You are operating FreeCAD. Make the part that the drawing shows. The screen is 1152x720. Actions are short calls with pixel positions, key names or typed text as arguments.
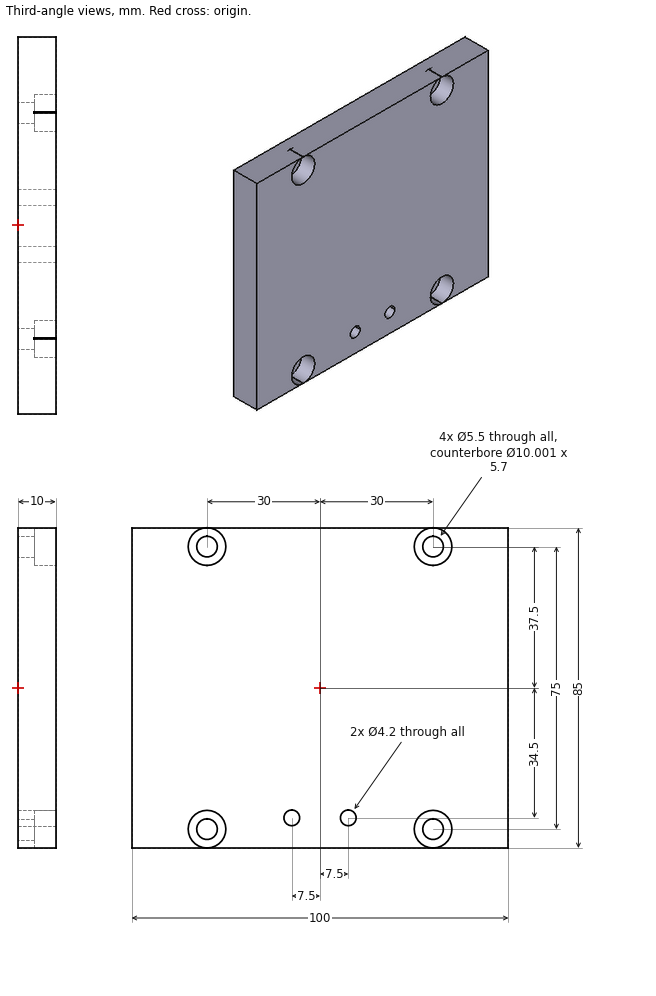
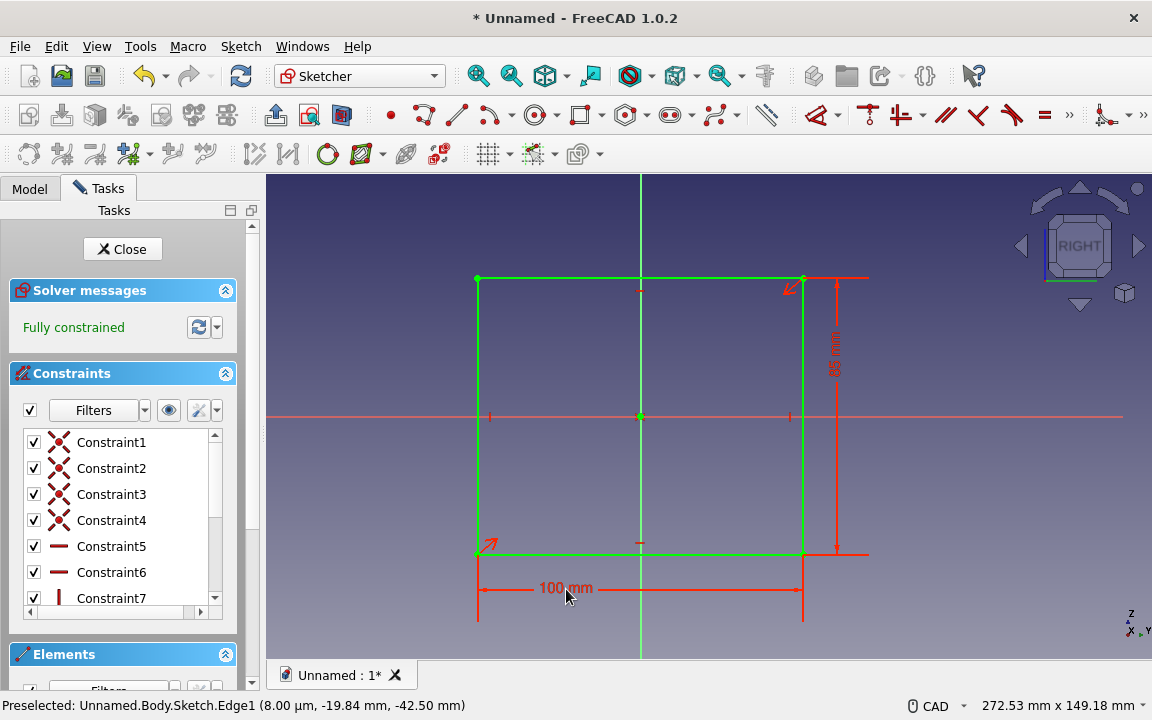
click(123, 249)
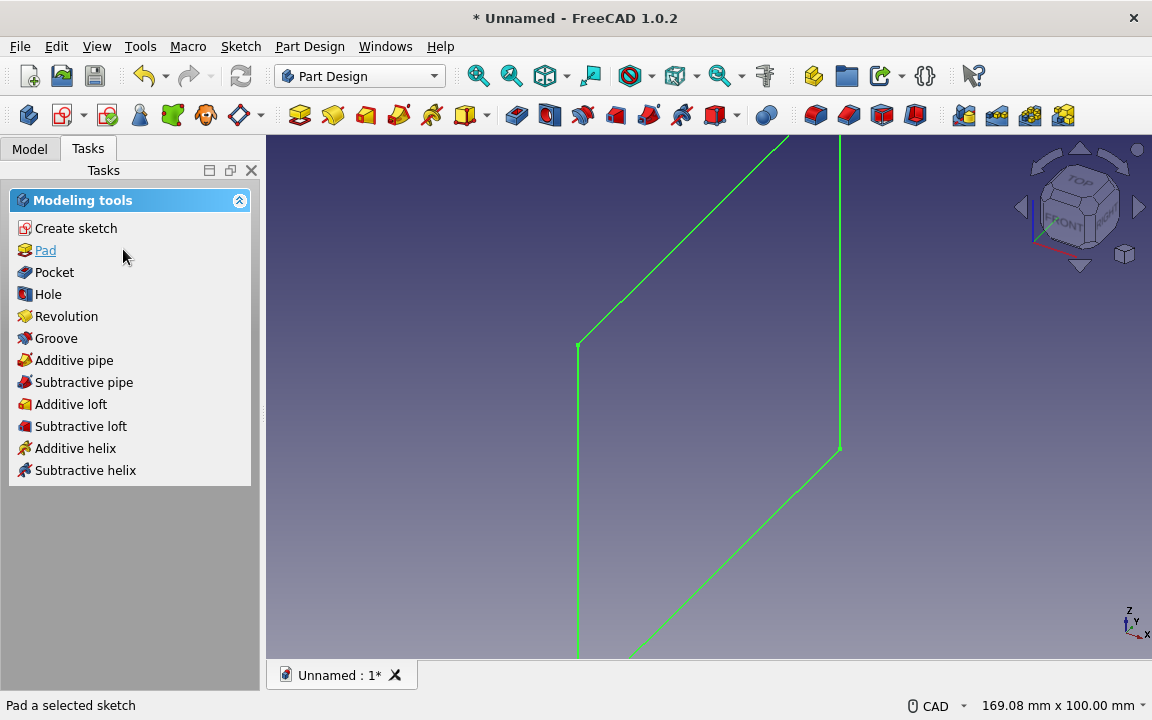
click(300, 116)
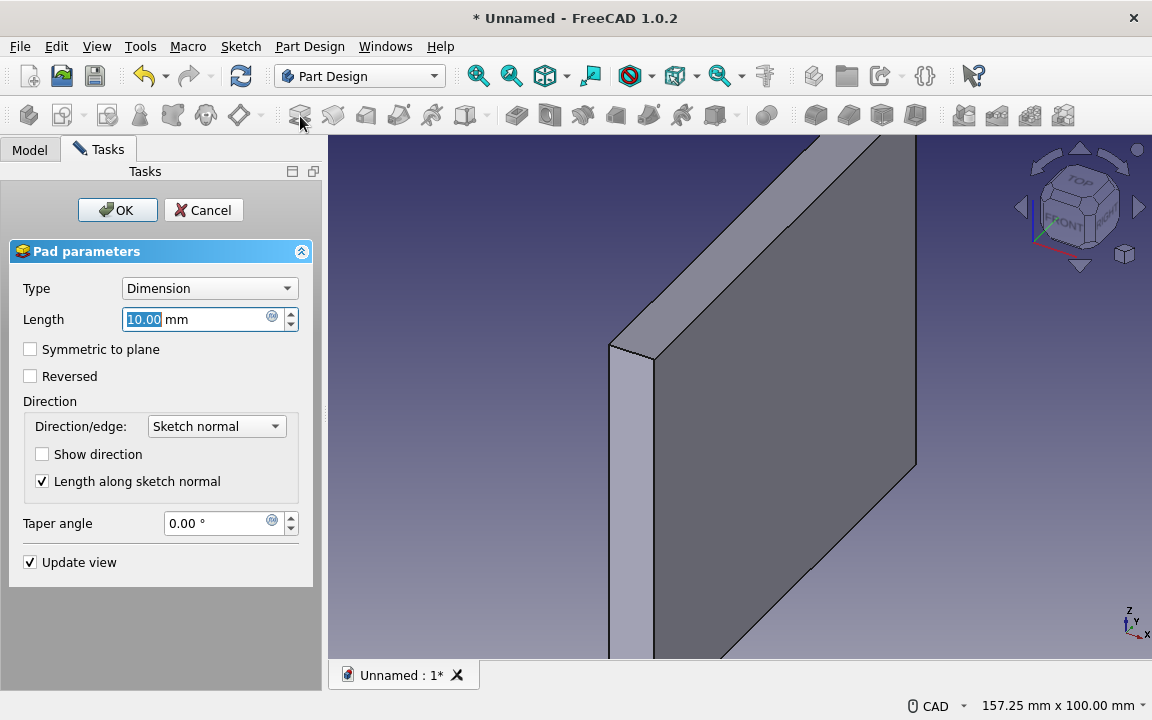
text(10)
key(Tab)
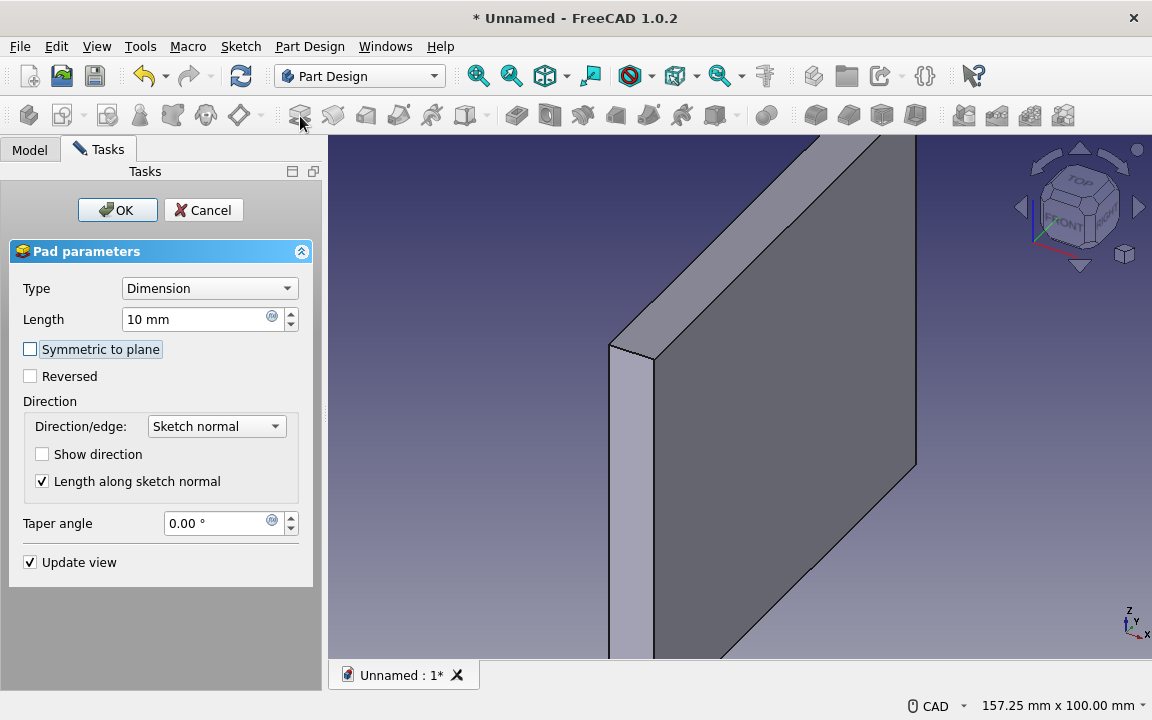
click(118, 210)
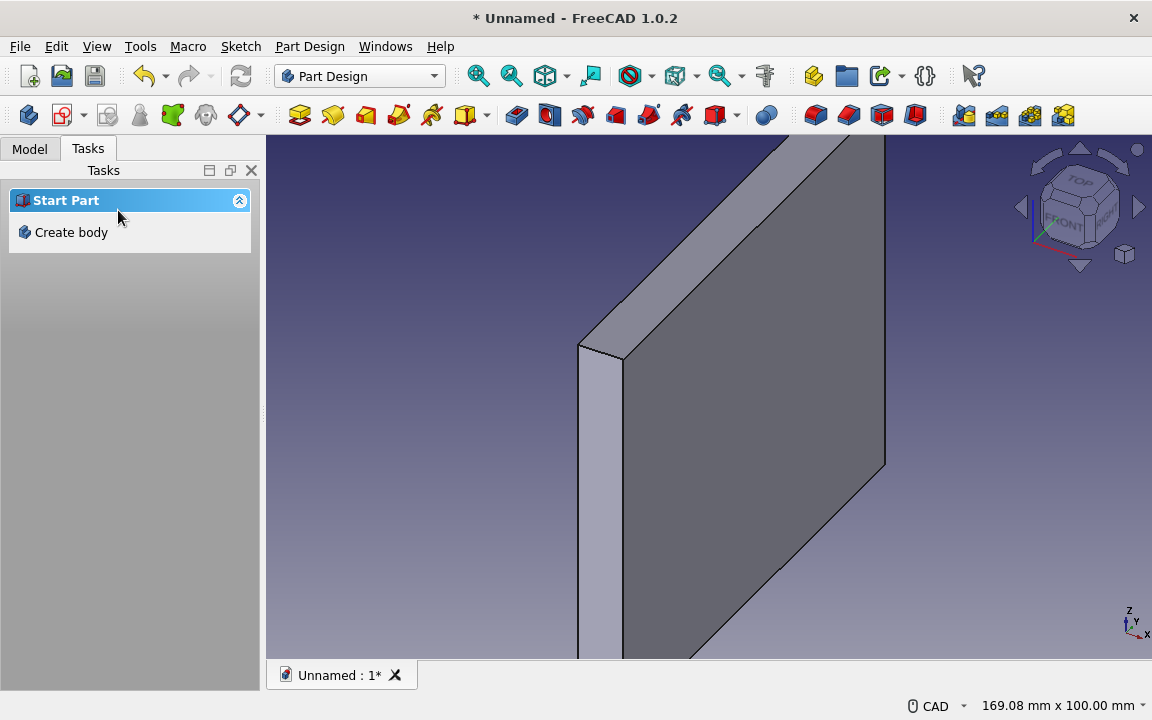
key(v)
key(f)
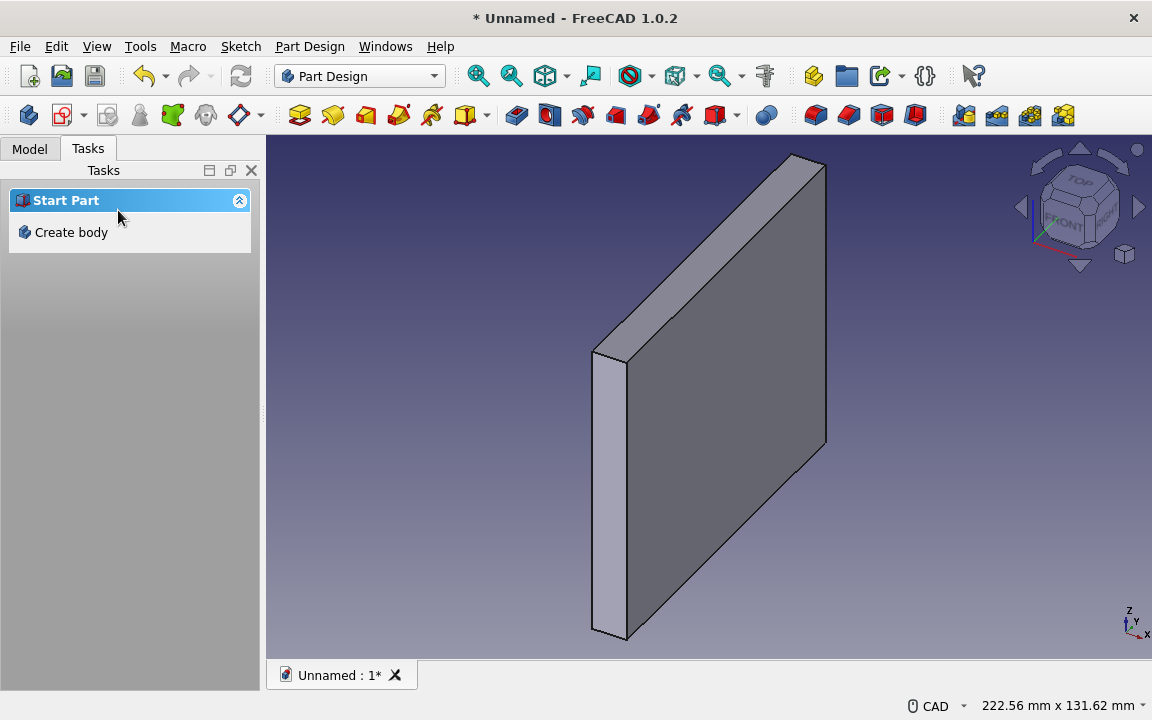
click(726, 402)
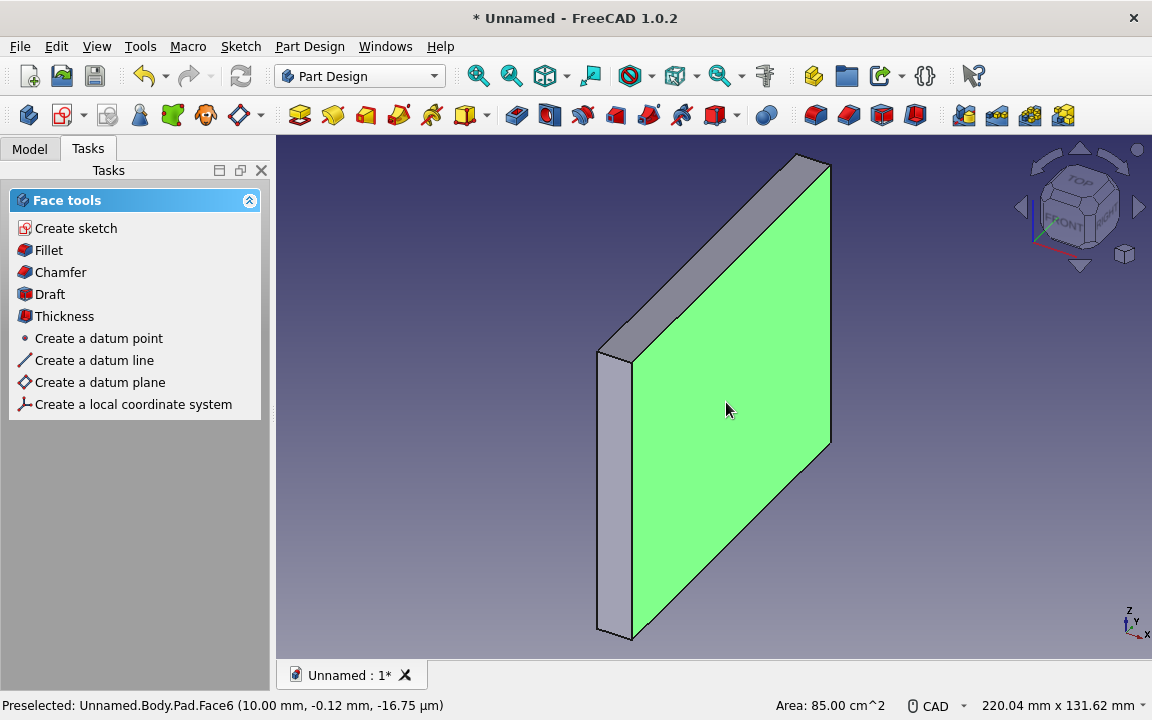
click(62, 116)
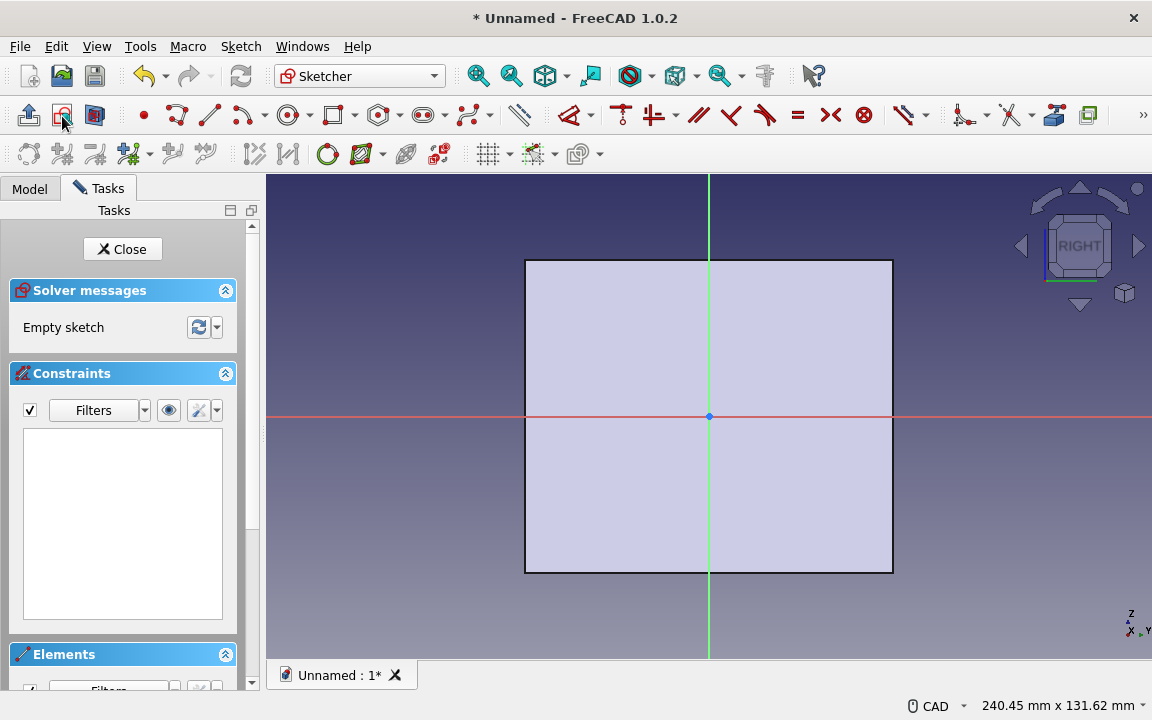
key(g)
key(c)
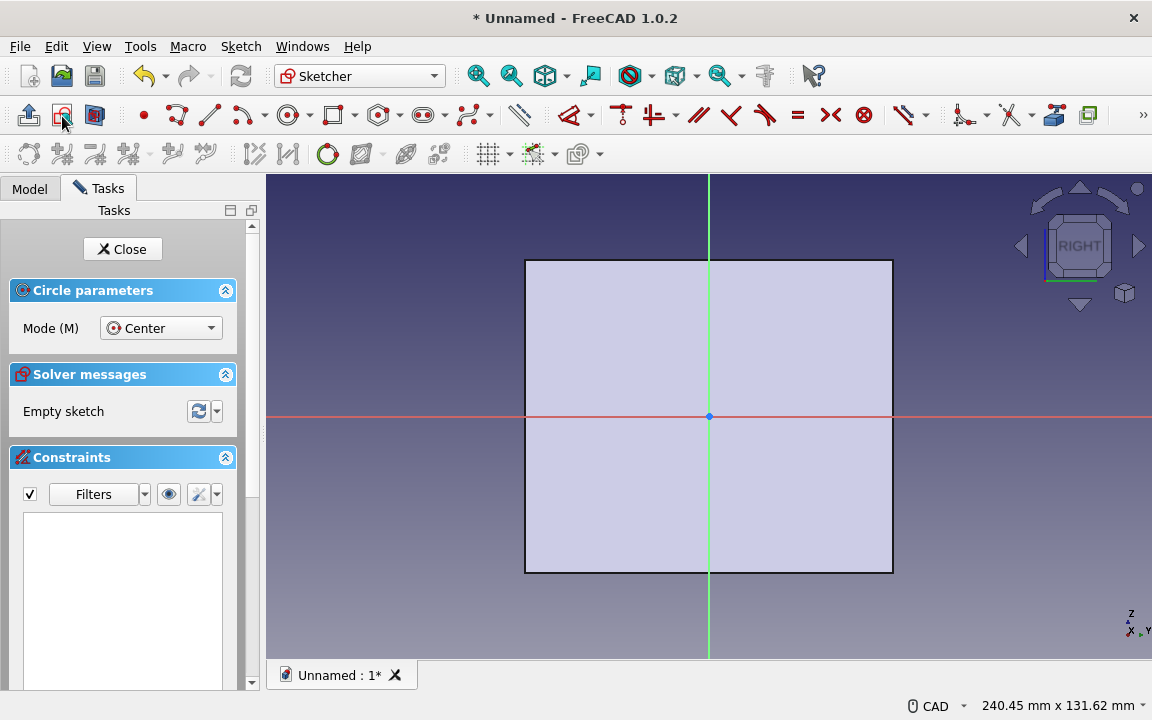
scroll(820, 278, up, 5)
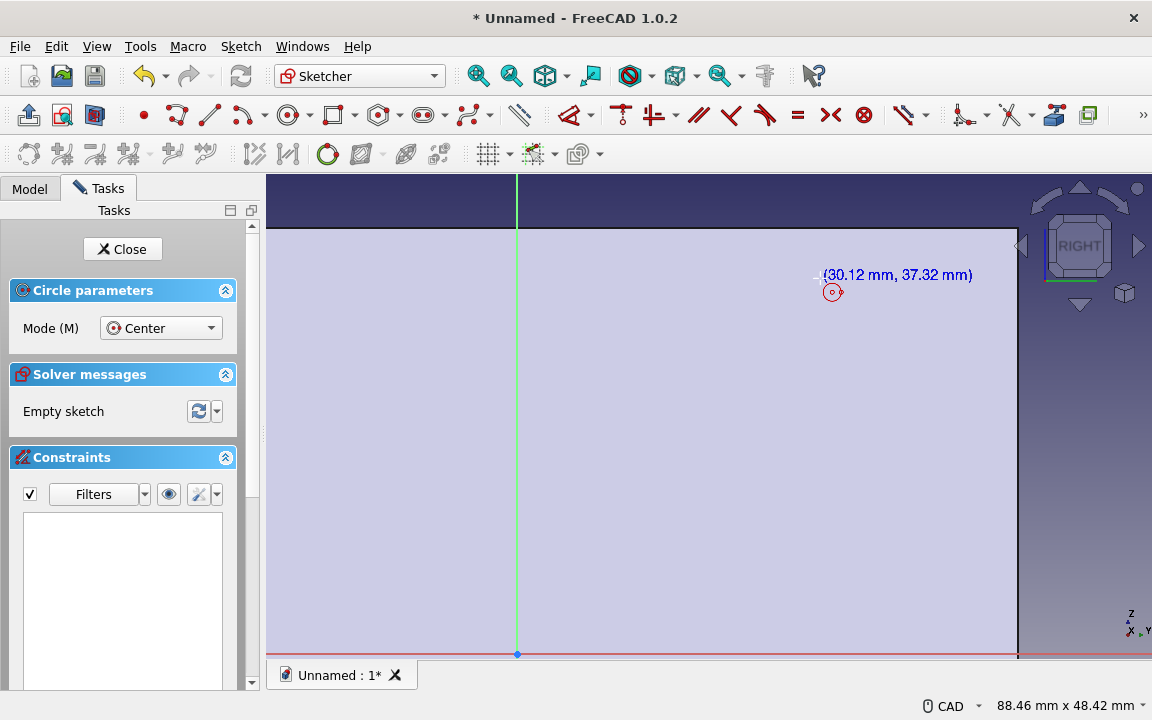
click(818, 279)
click(837, 259)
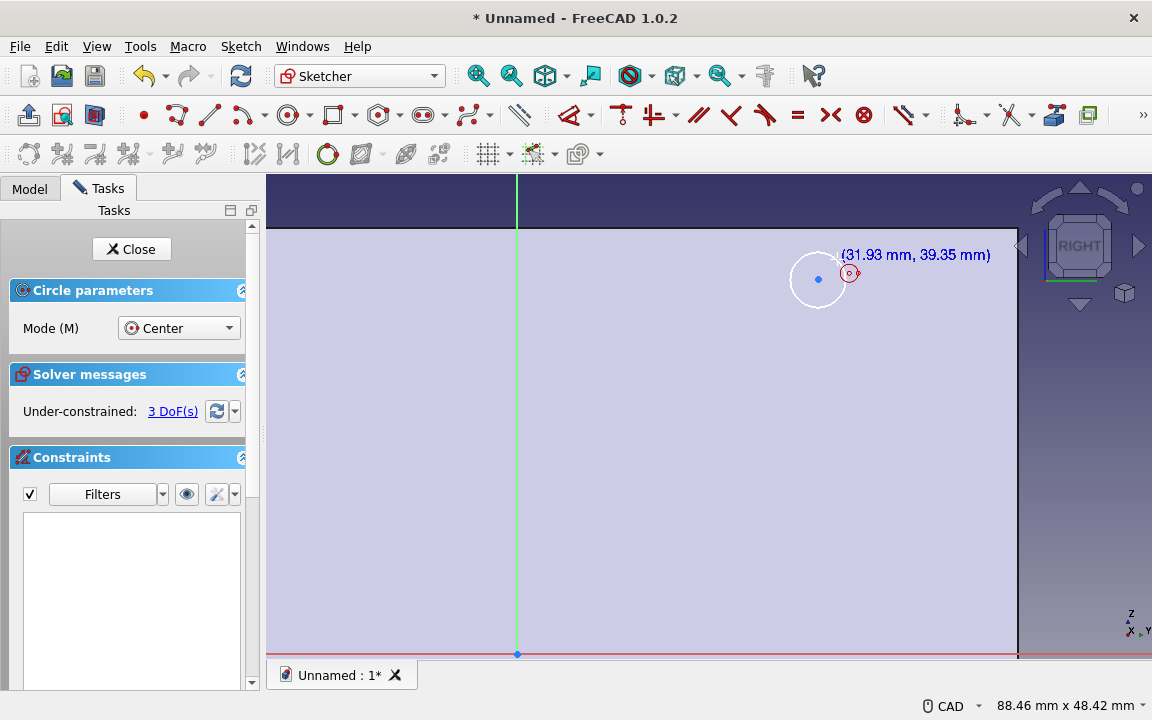
scroll(712, 278, down, 5)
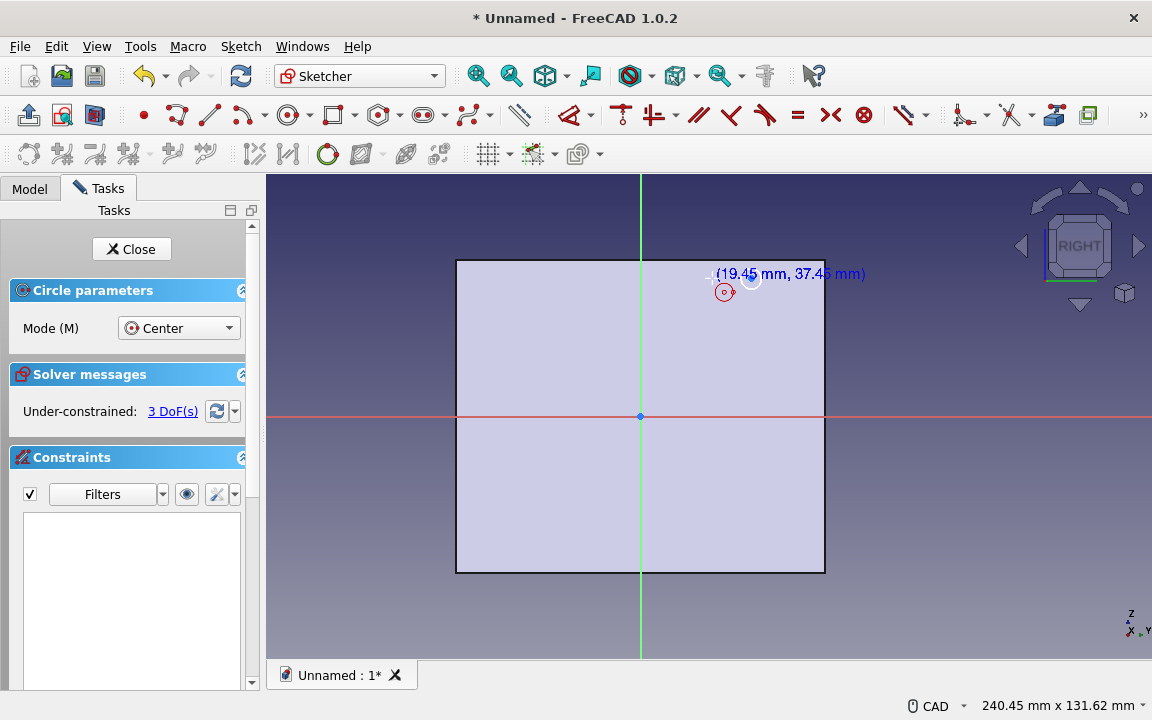
scroll(530, 278, up, 5)